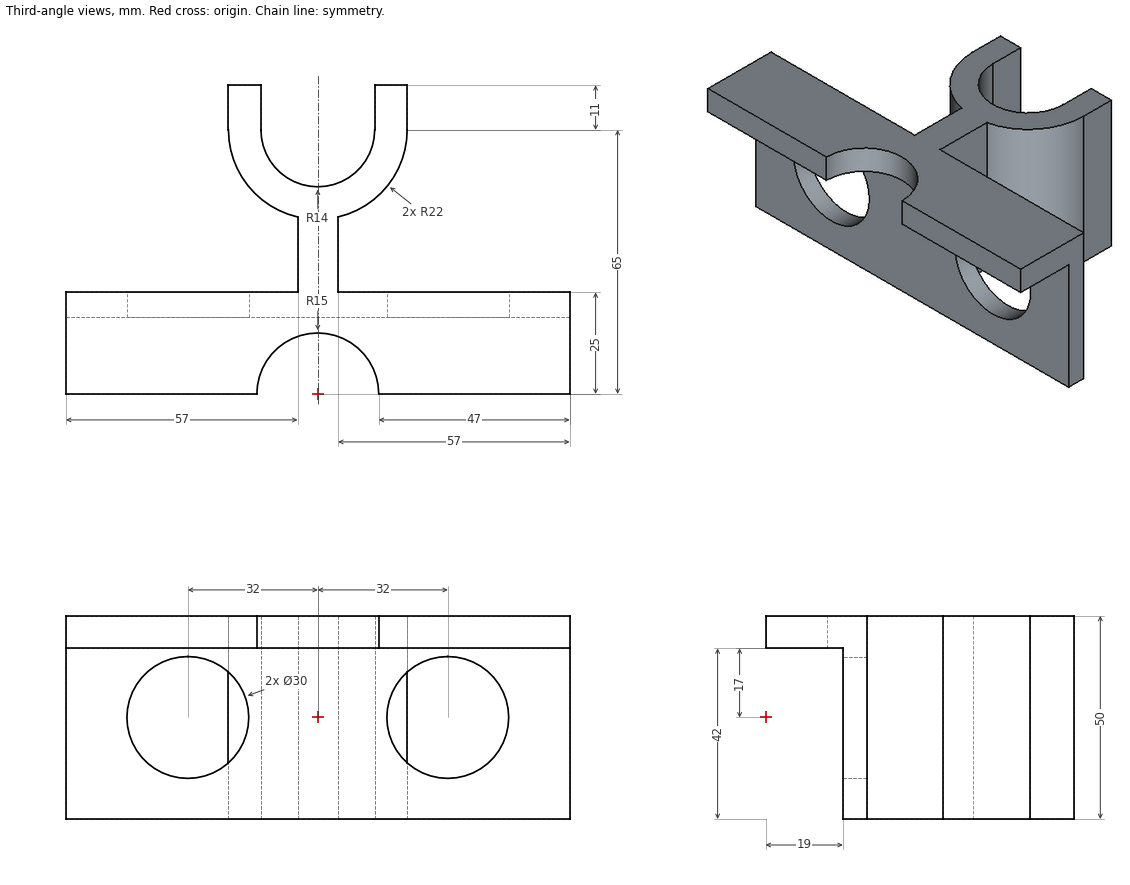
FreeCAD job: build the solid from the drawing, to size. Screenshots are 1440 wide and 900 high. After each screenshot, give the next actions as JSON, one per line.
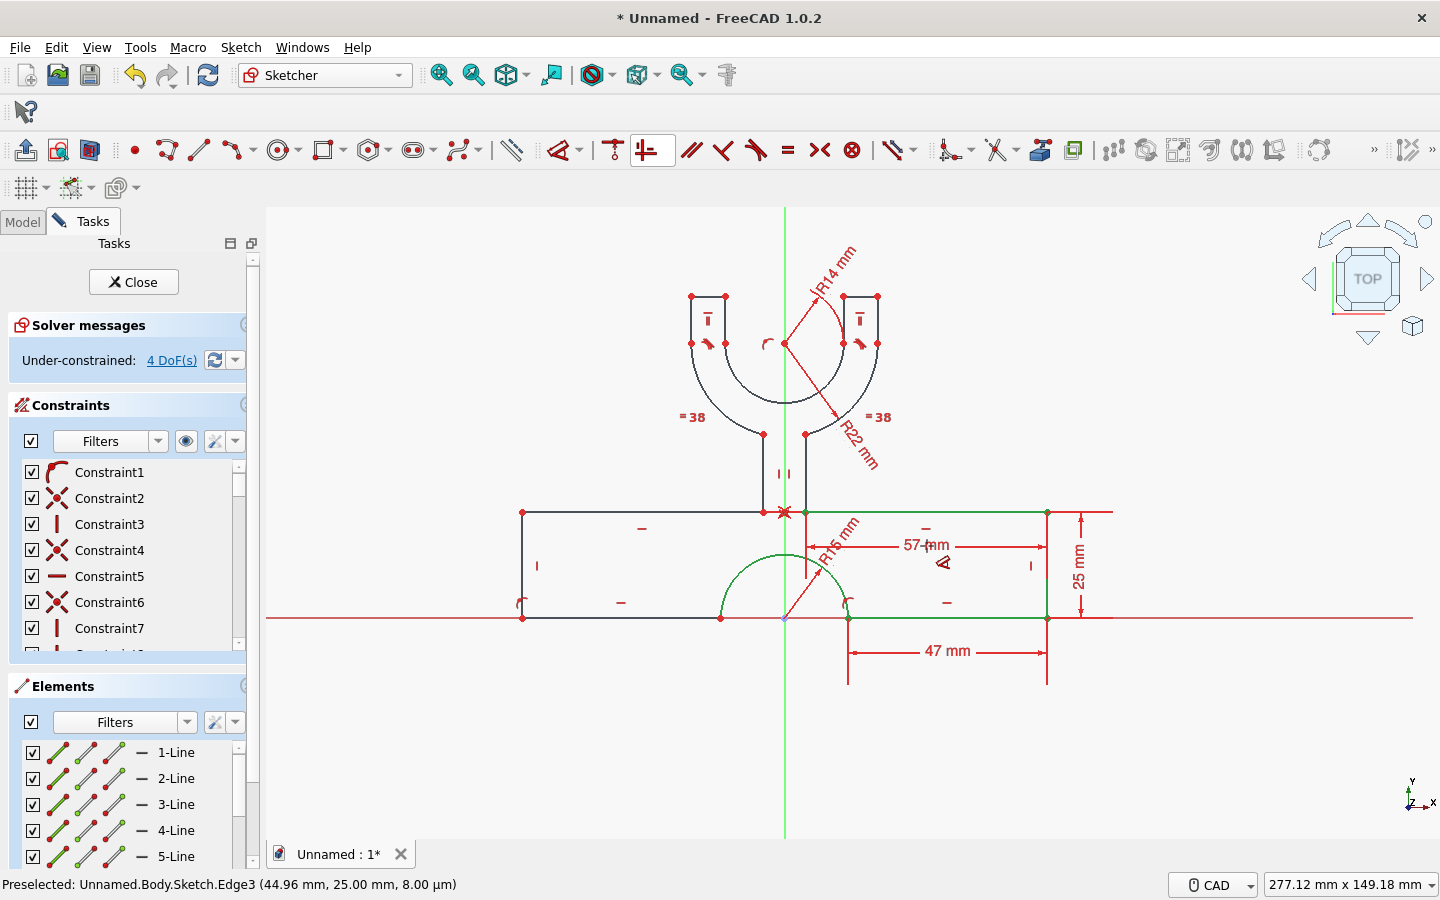
{"action": "left_click", "coordinate": [878, 330]}
{"action": "left_click", "coordinate": [912, 320]}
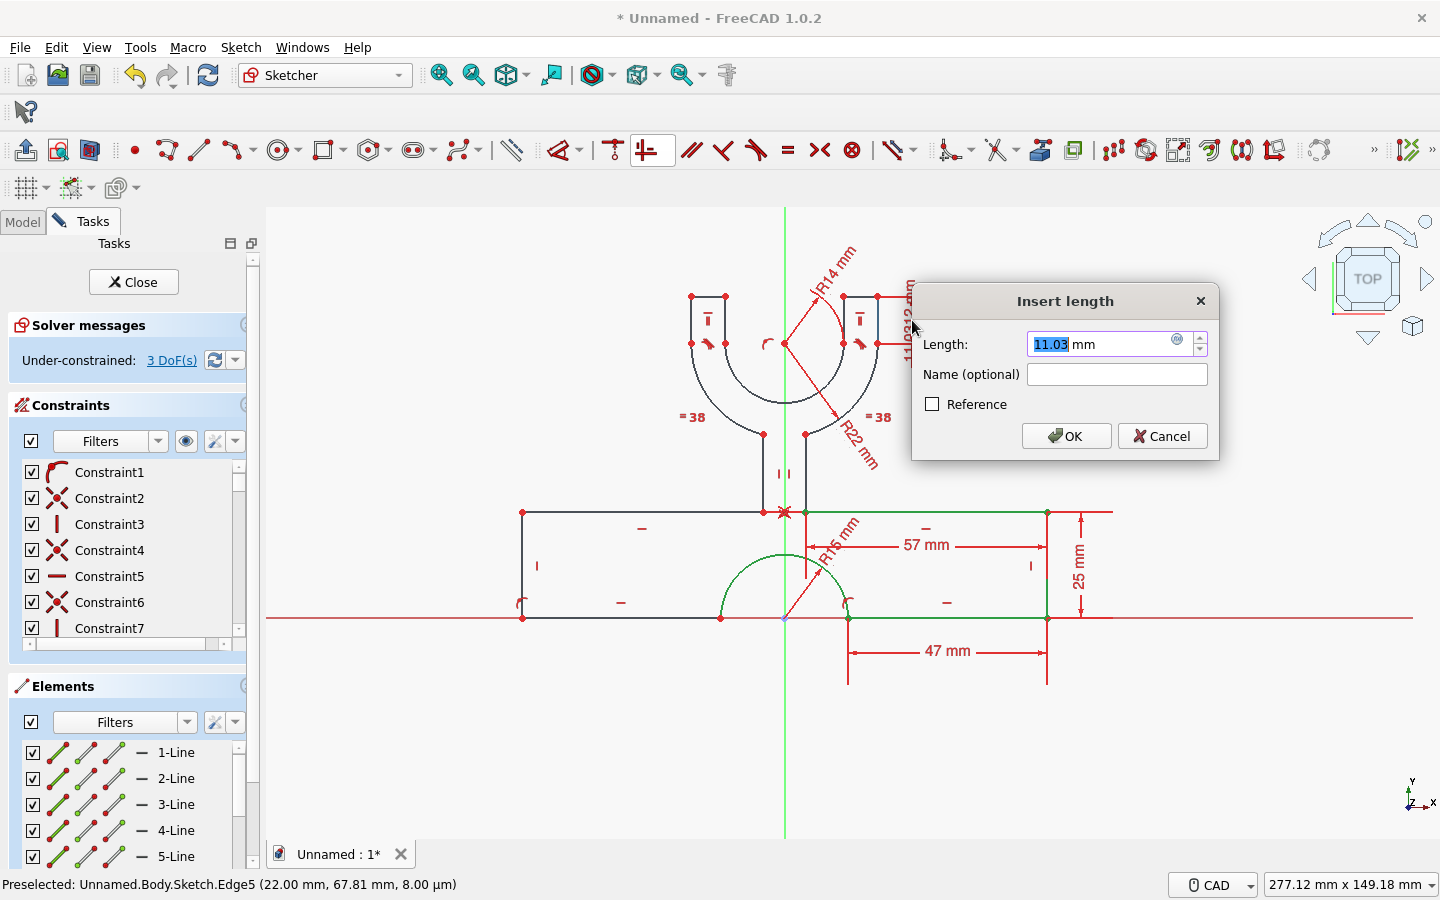
{"action": "type", "text": "11"}
{"action": "key", "text": "Return"}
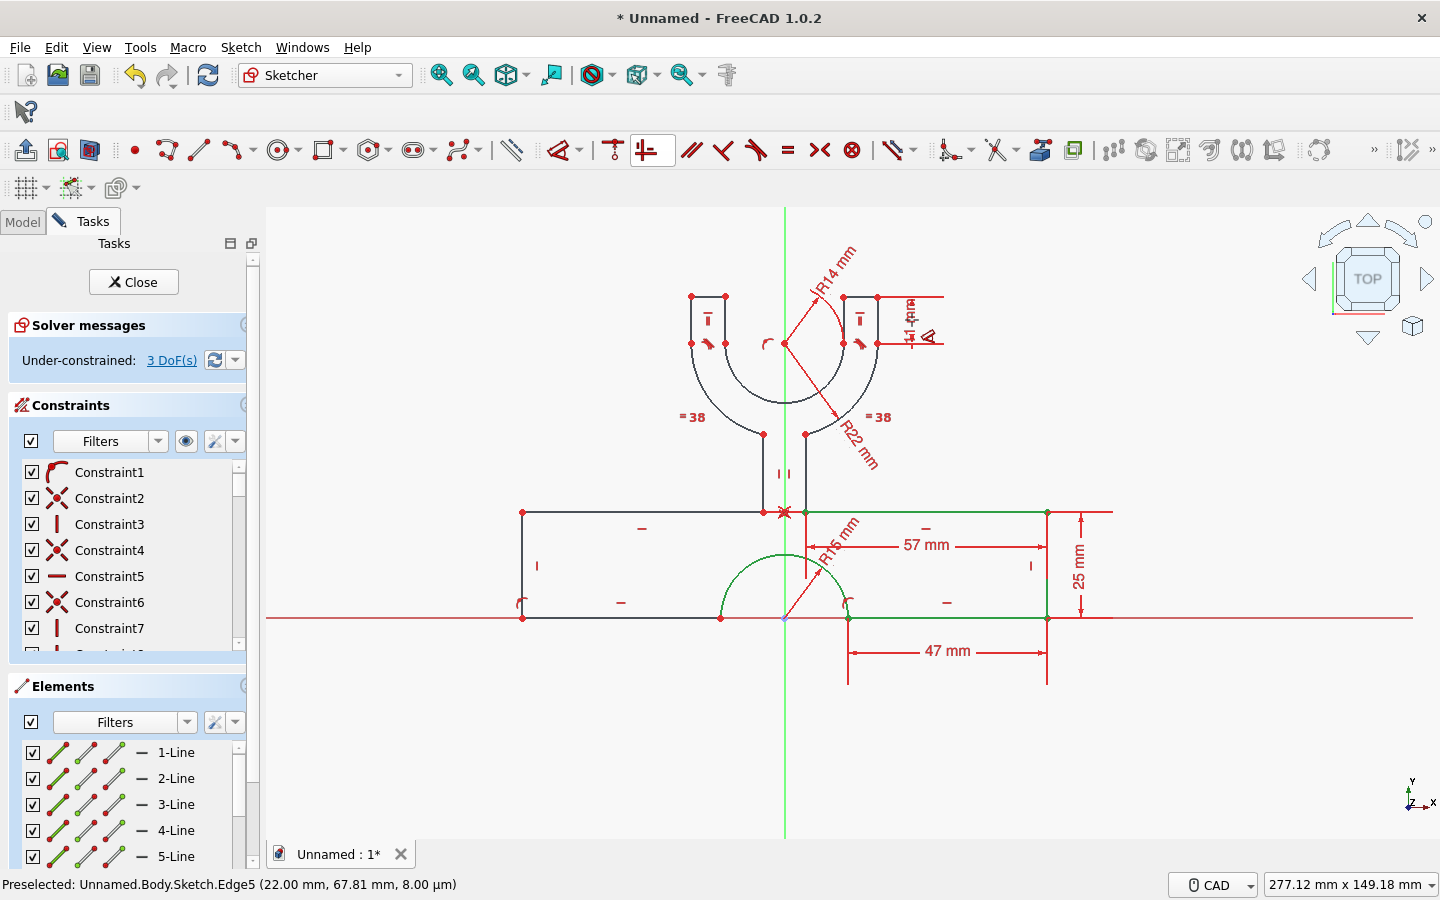
{"action": "left_click", "coordinate": [725, 330]}
{"action": "left_click", "coordinate": [759, 320]}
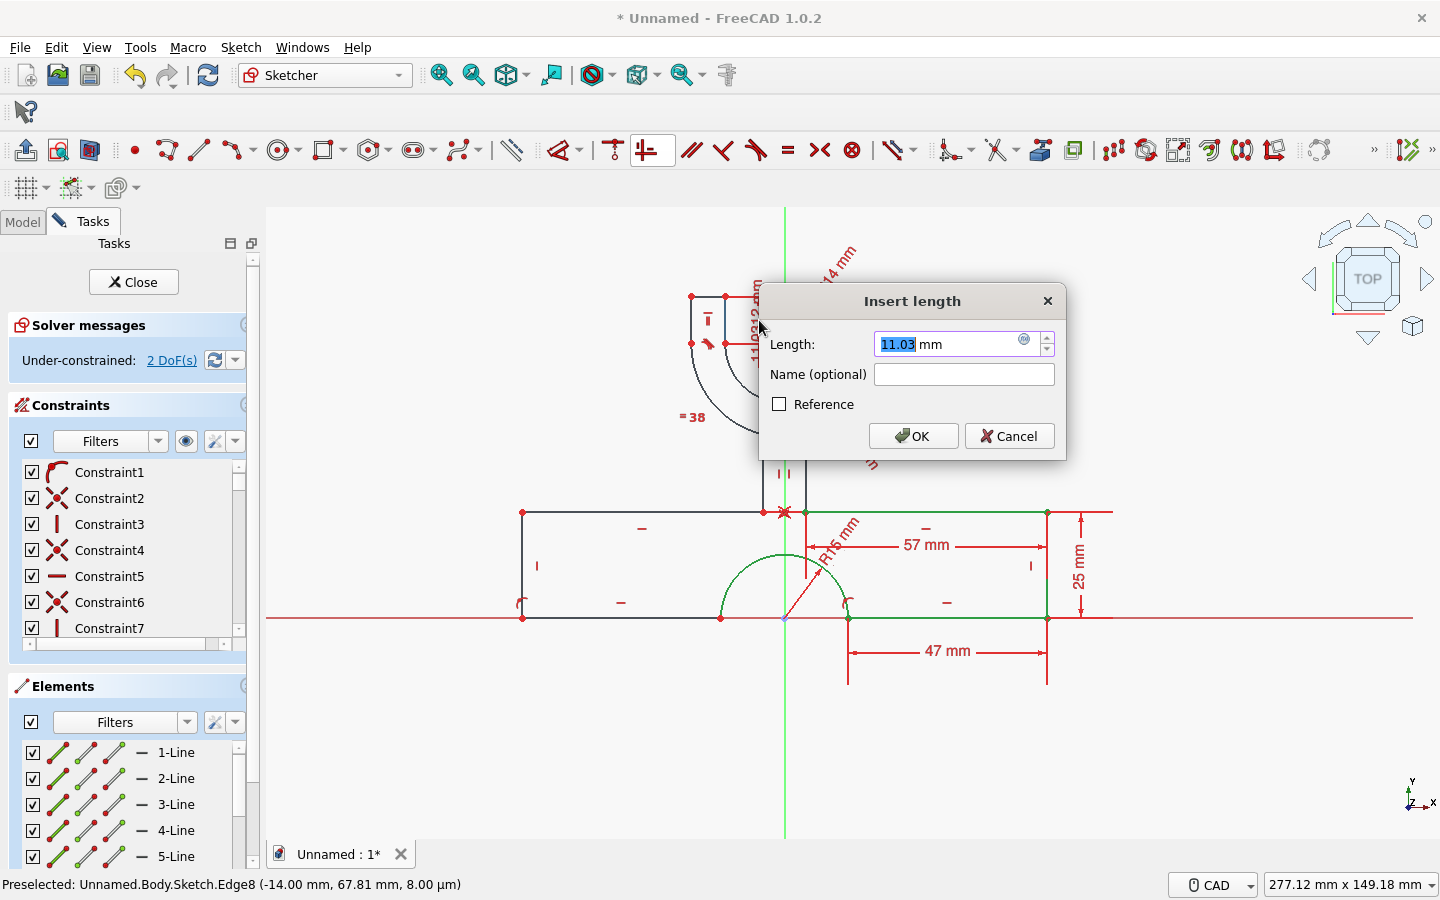
{"action": "type", "text": "11"}
{"action": "key", "text": "Return"}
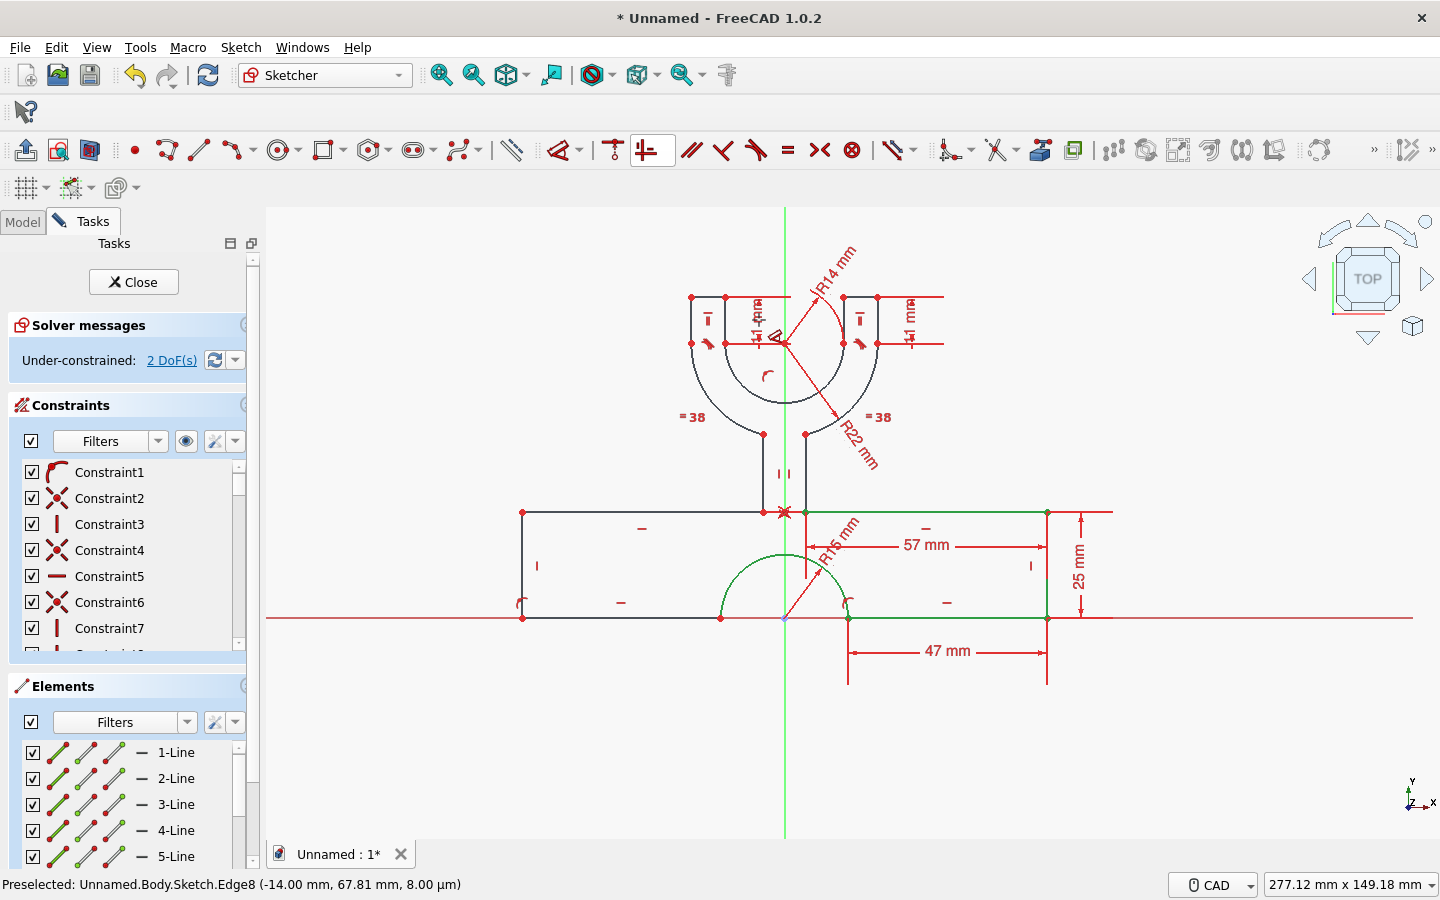
{"action": "left_click", "coordinate": [691, 512]}
{"action": "left_click", "coordinate": [643, 546]}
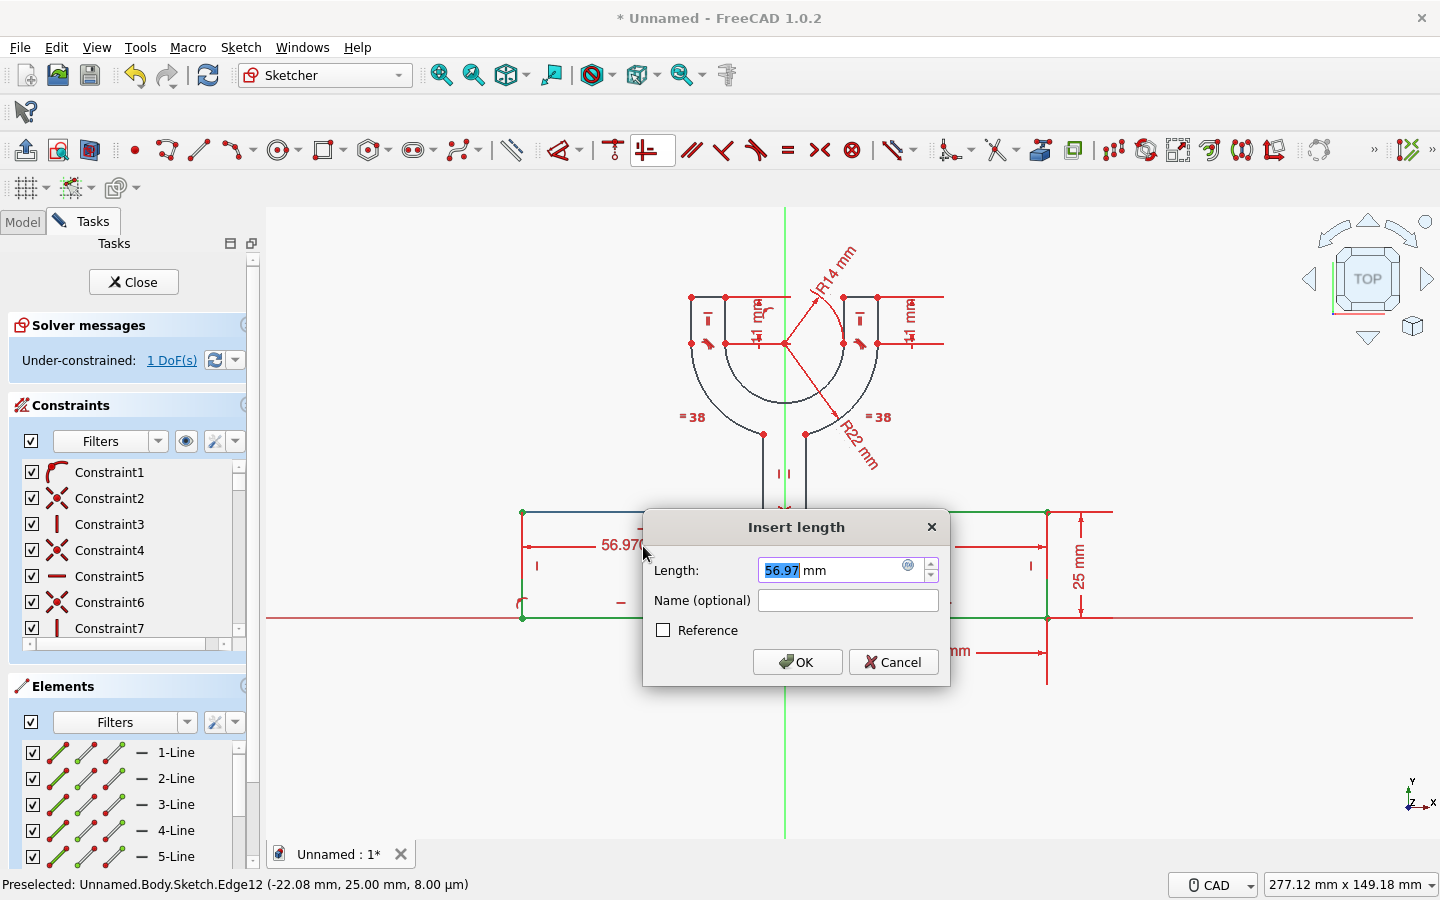
{"action": "type", "text": "57"}
{"action": "key", "text": "Return"}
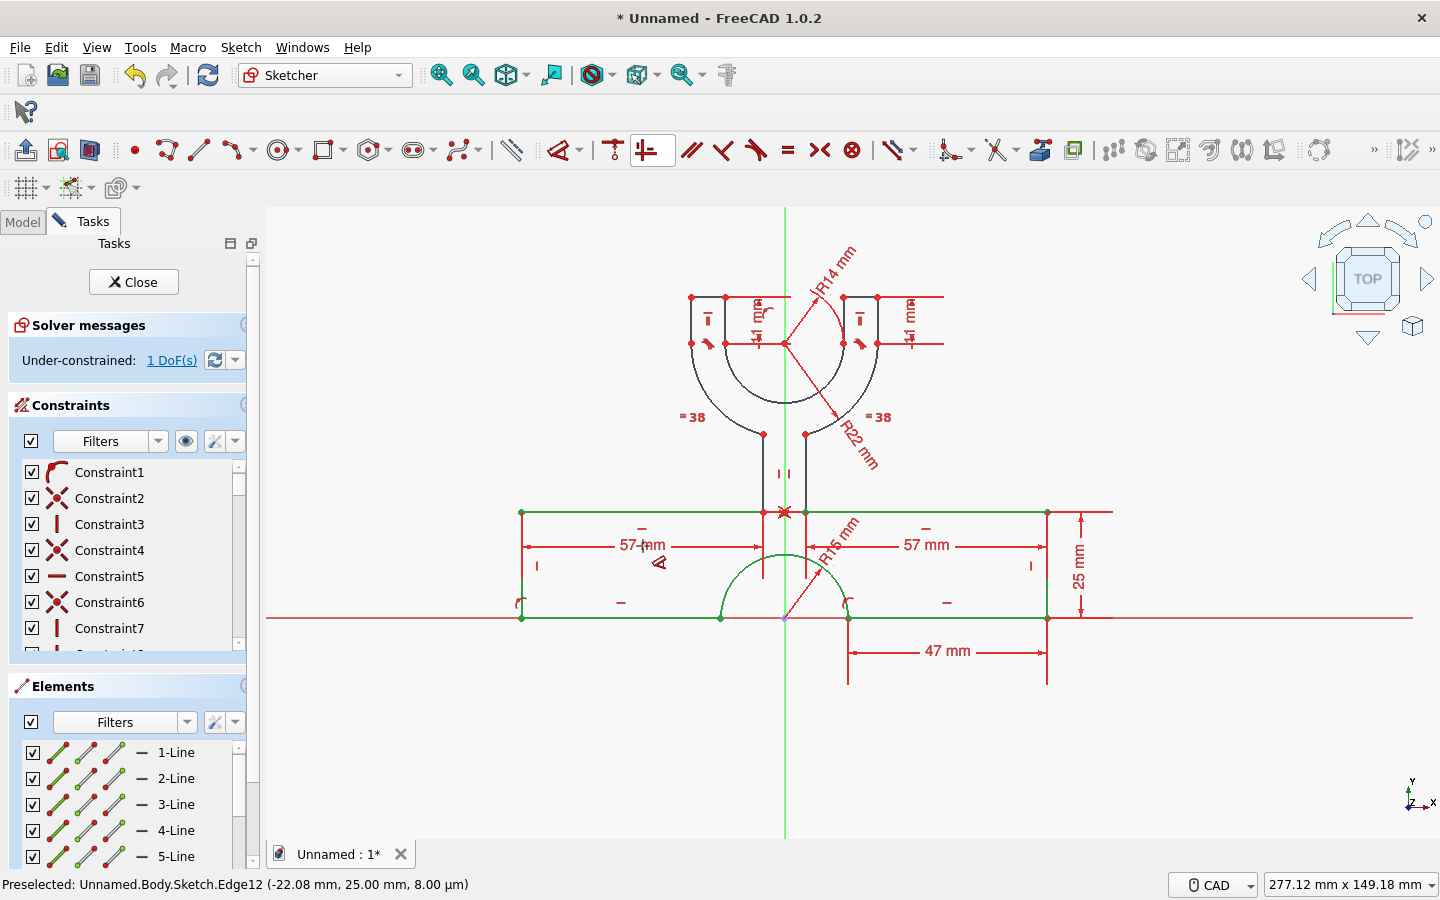
{"action": "left_click", "coordinate": [878, 344]}
{"action": "left_click", "coordinate": [912, 481]}